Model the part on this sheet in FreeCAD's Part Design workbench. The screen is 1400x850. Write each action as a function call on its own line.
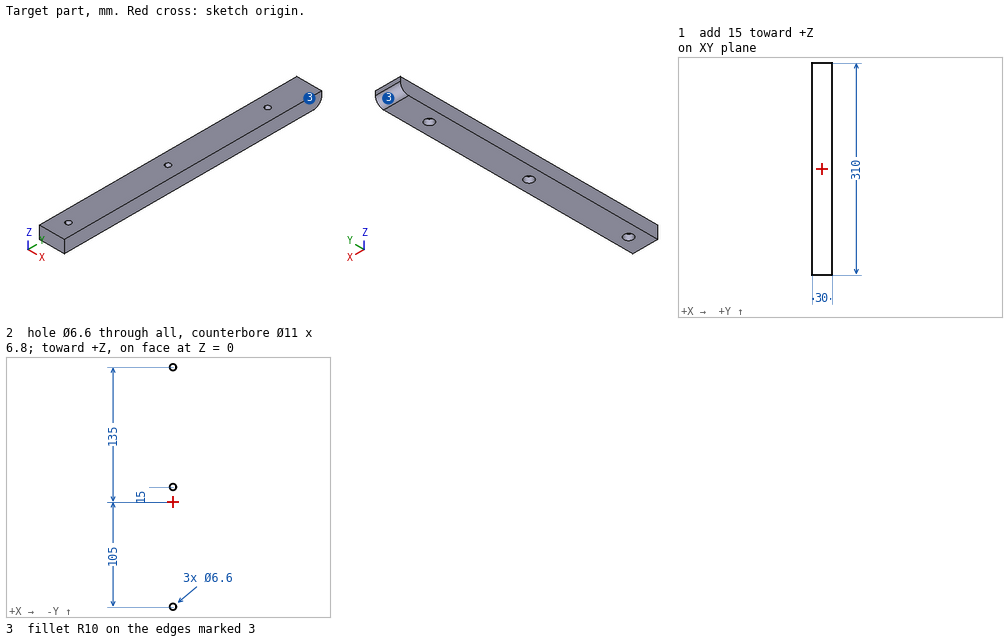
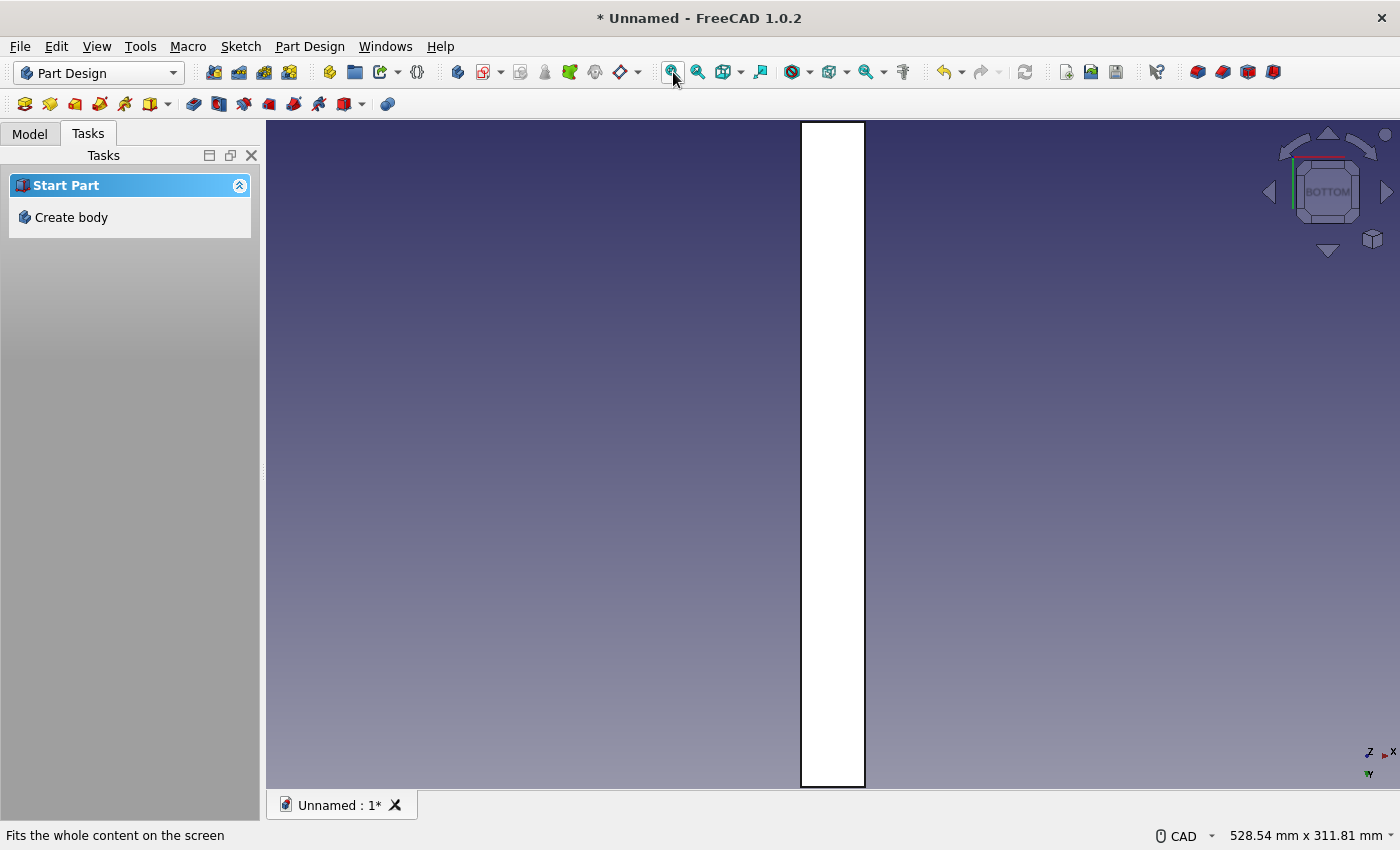
click(833, 739)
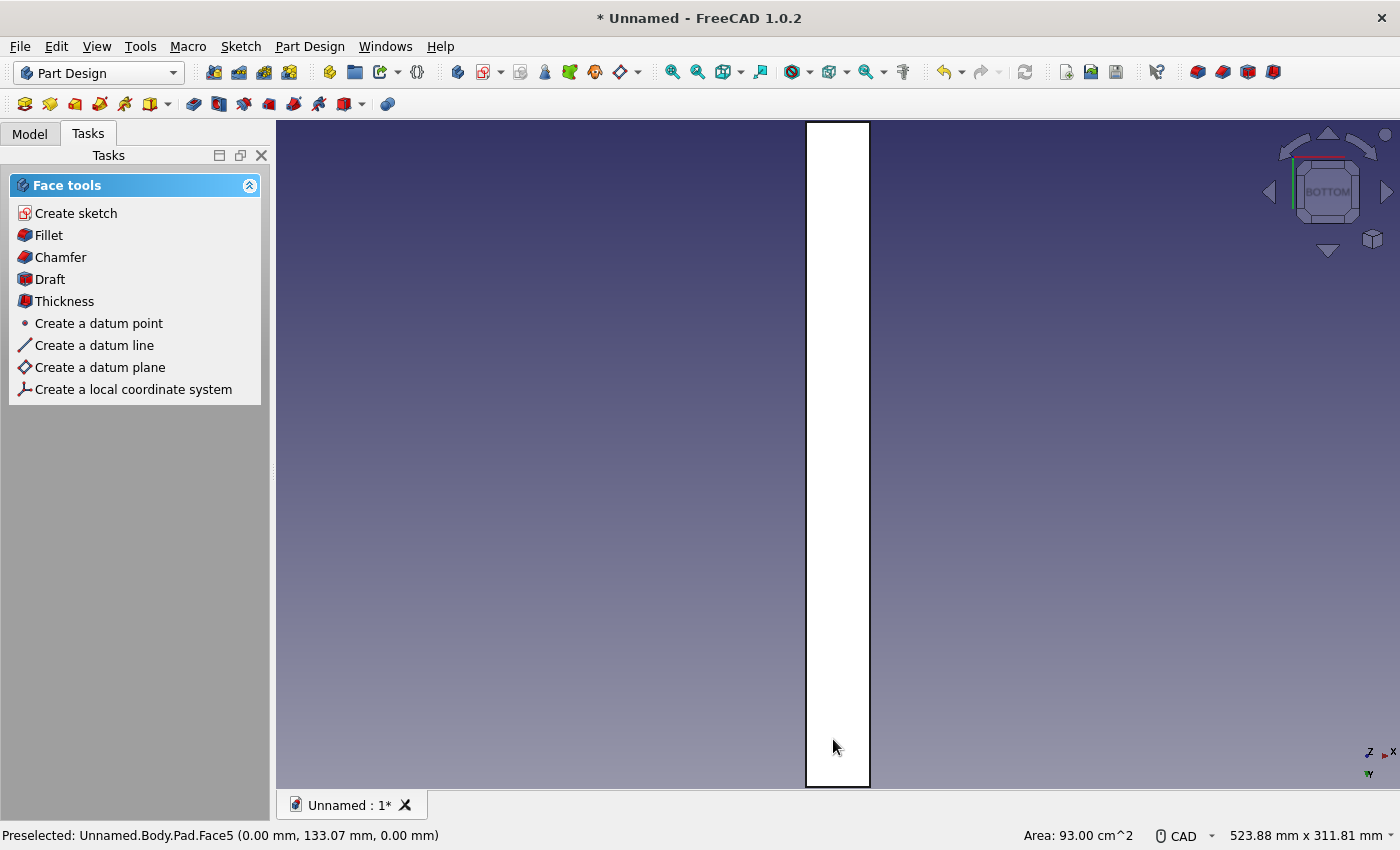
click(482, 72)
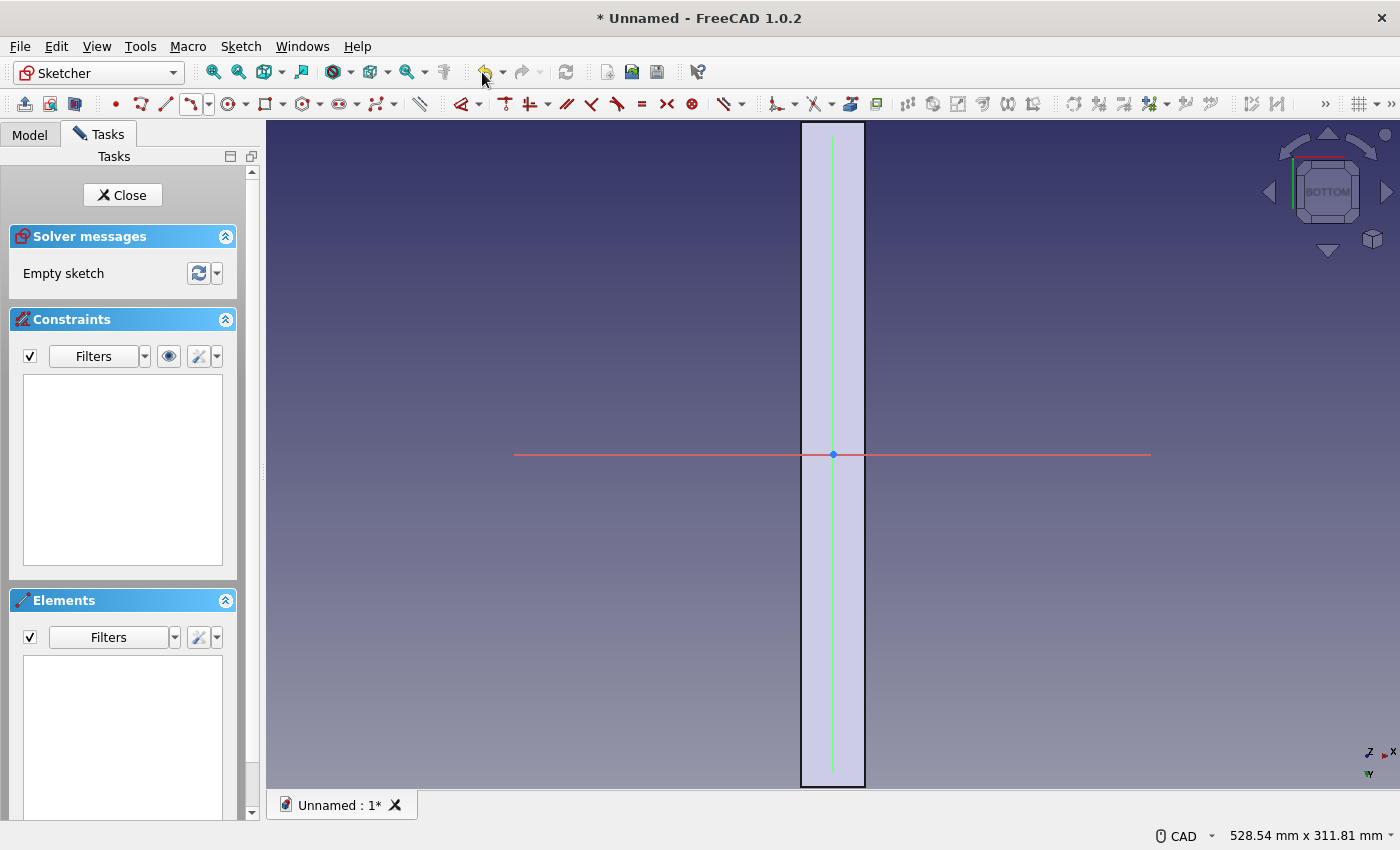
scroll(455, 600, down, 1)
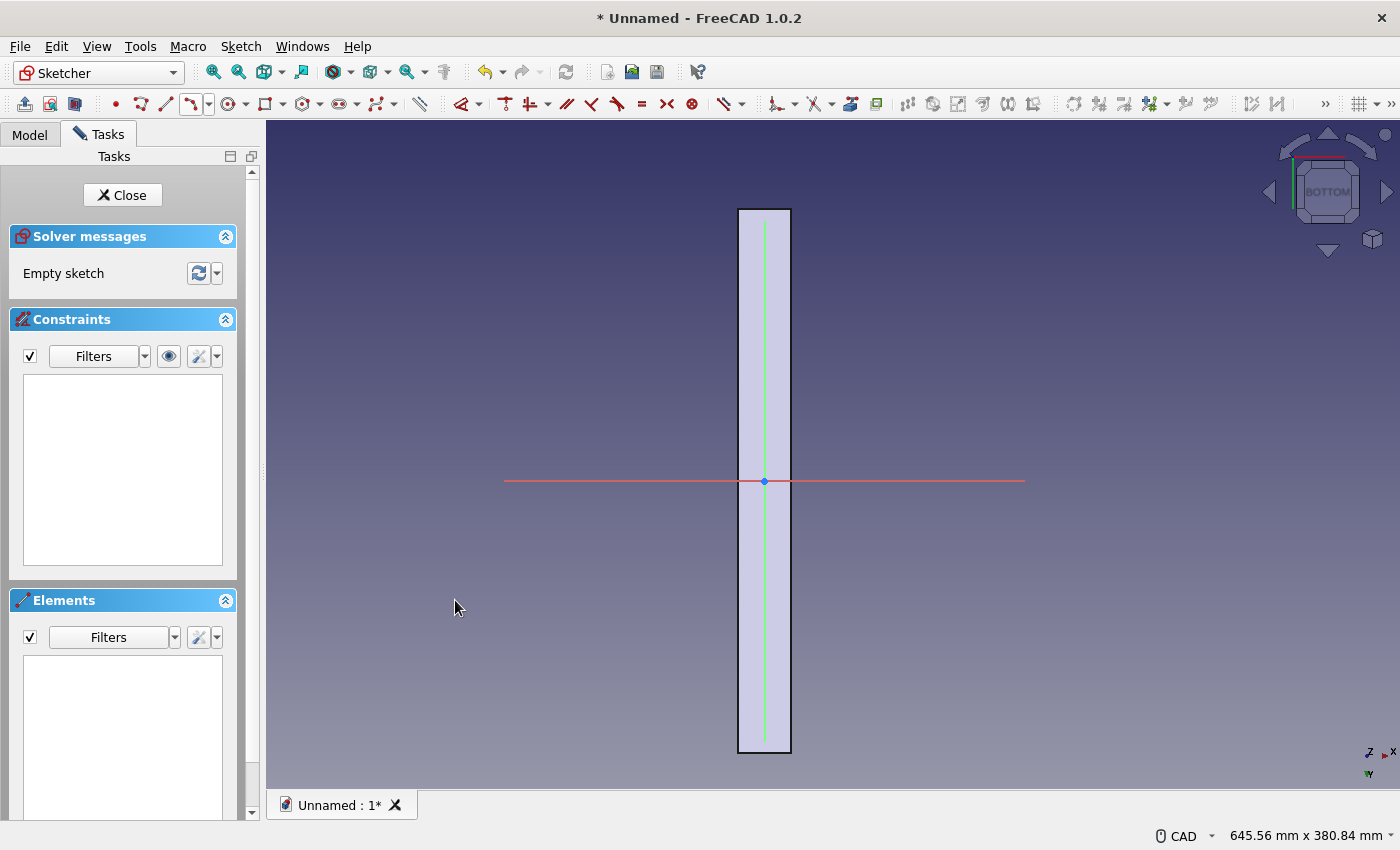
click(228, 104)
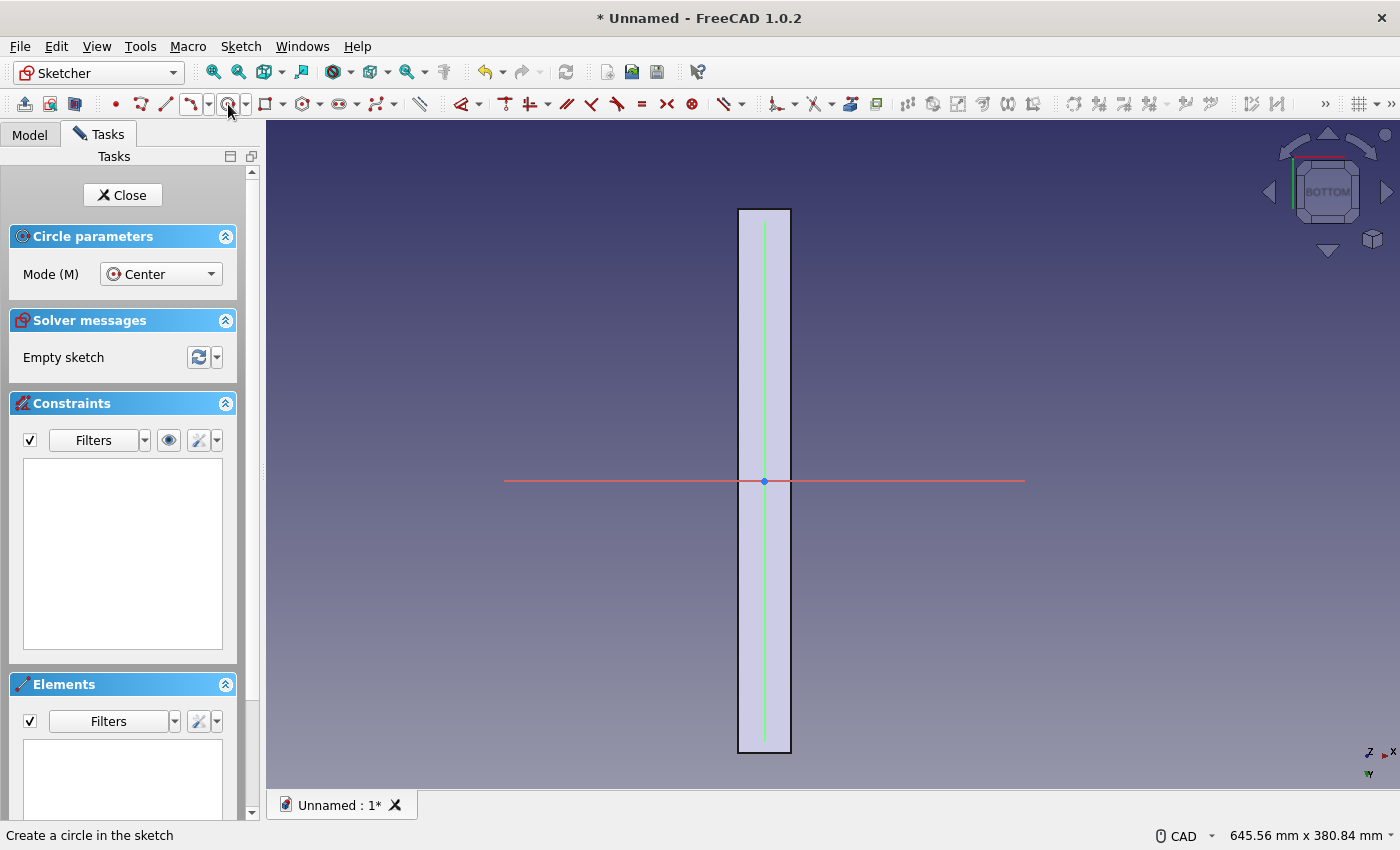
scroll(765, 665, up, 7)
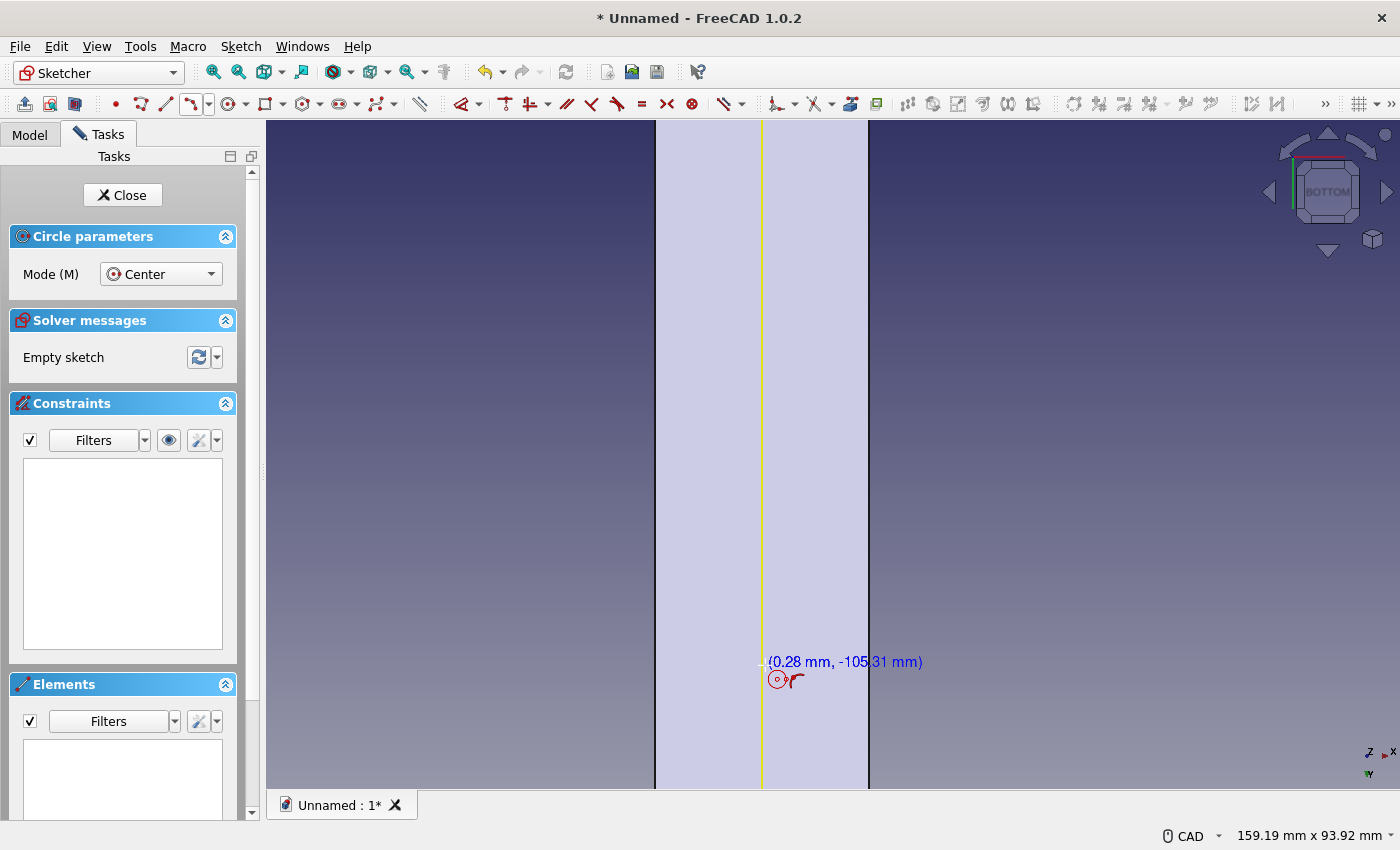
scroll(765, 666, down, 7)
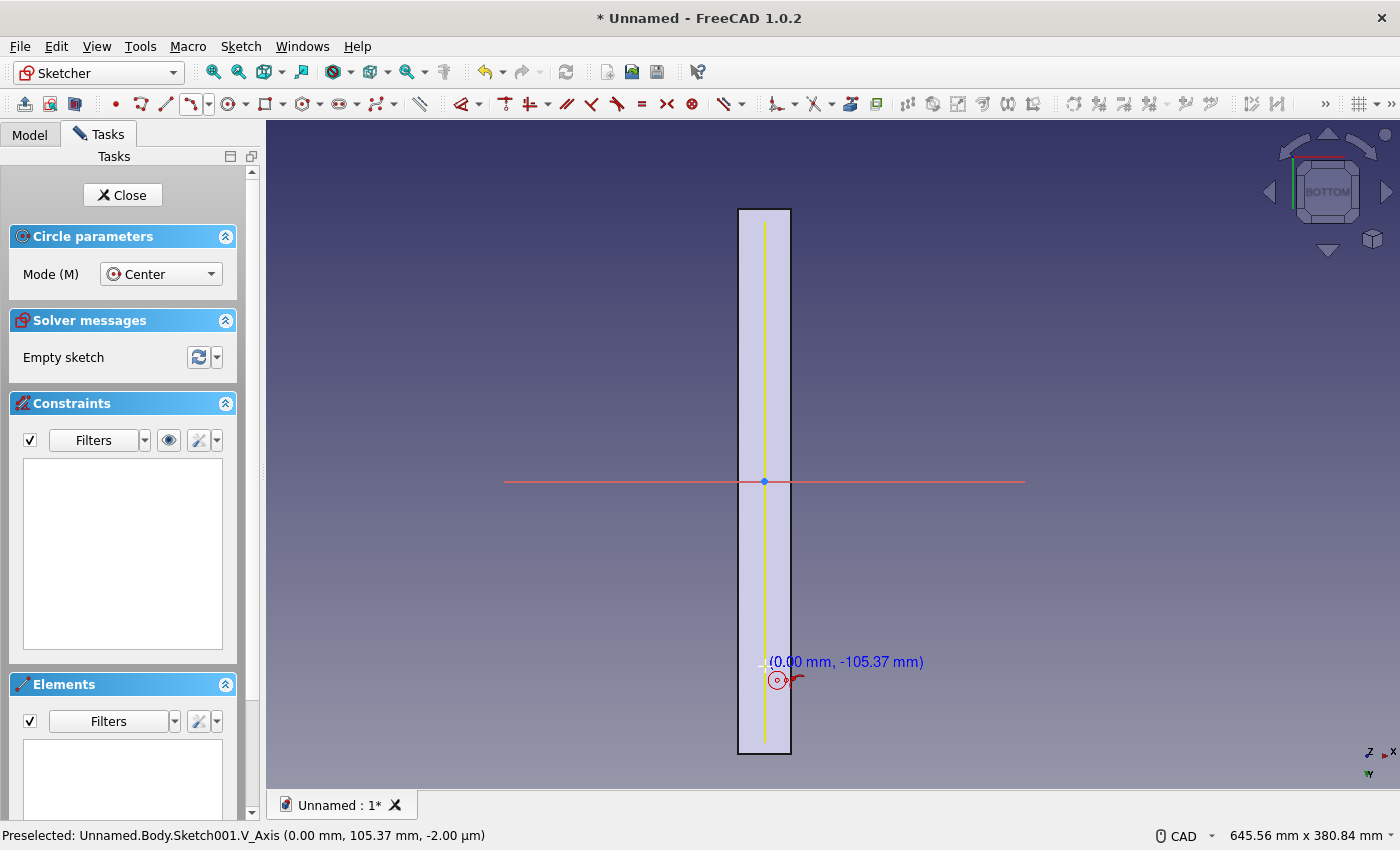
click(765, 666)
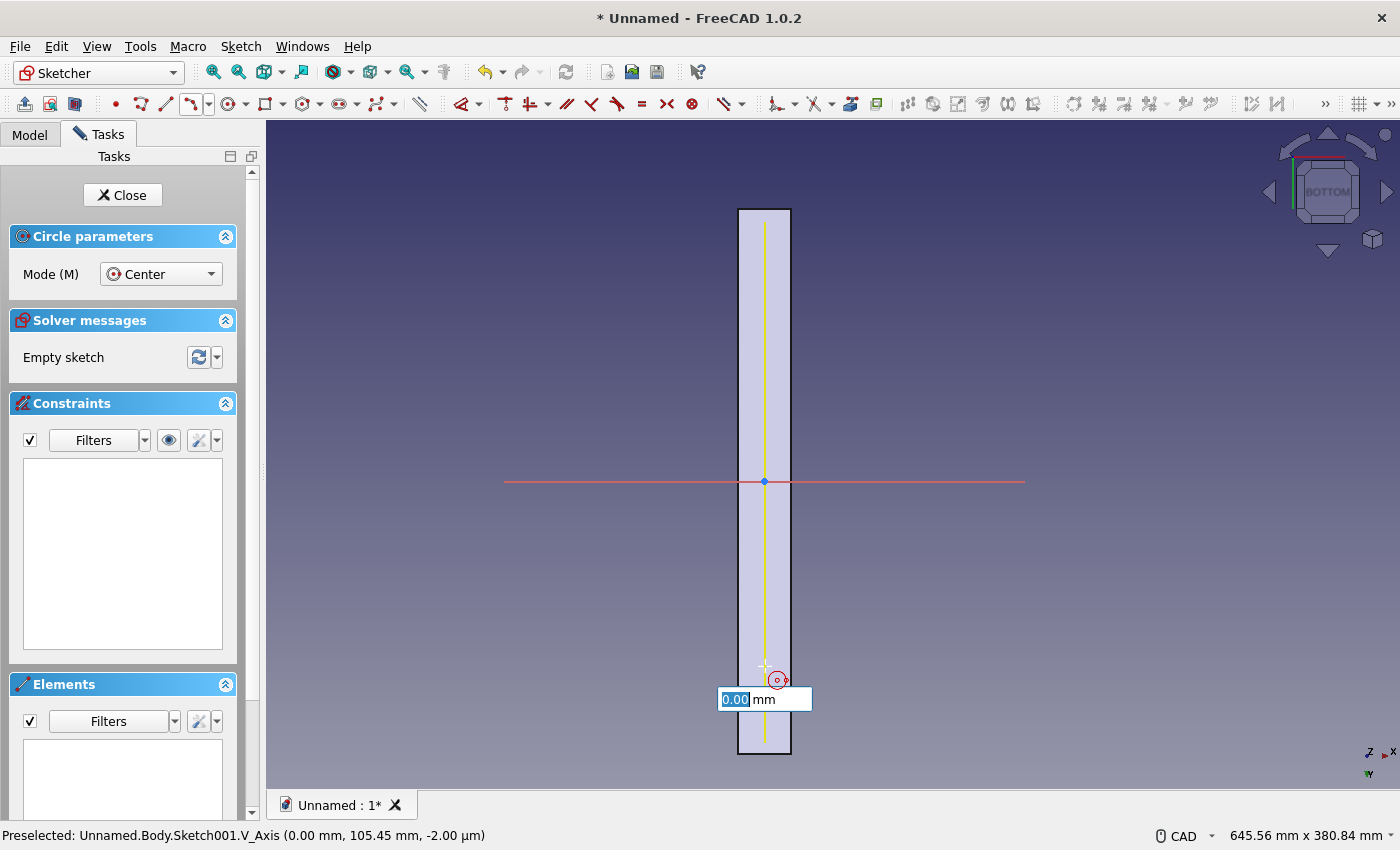
scroll(770, 664, up, 6)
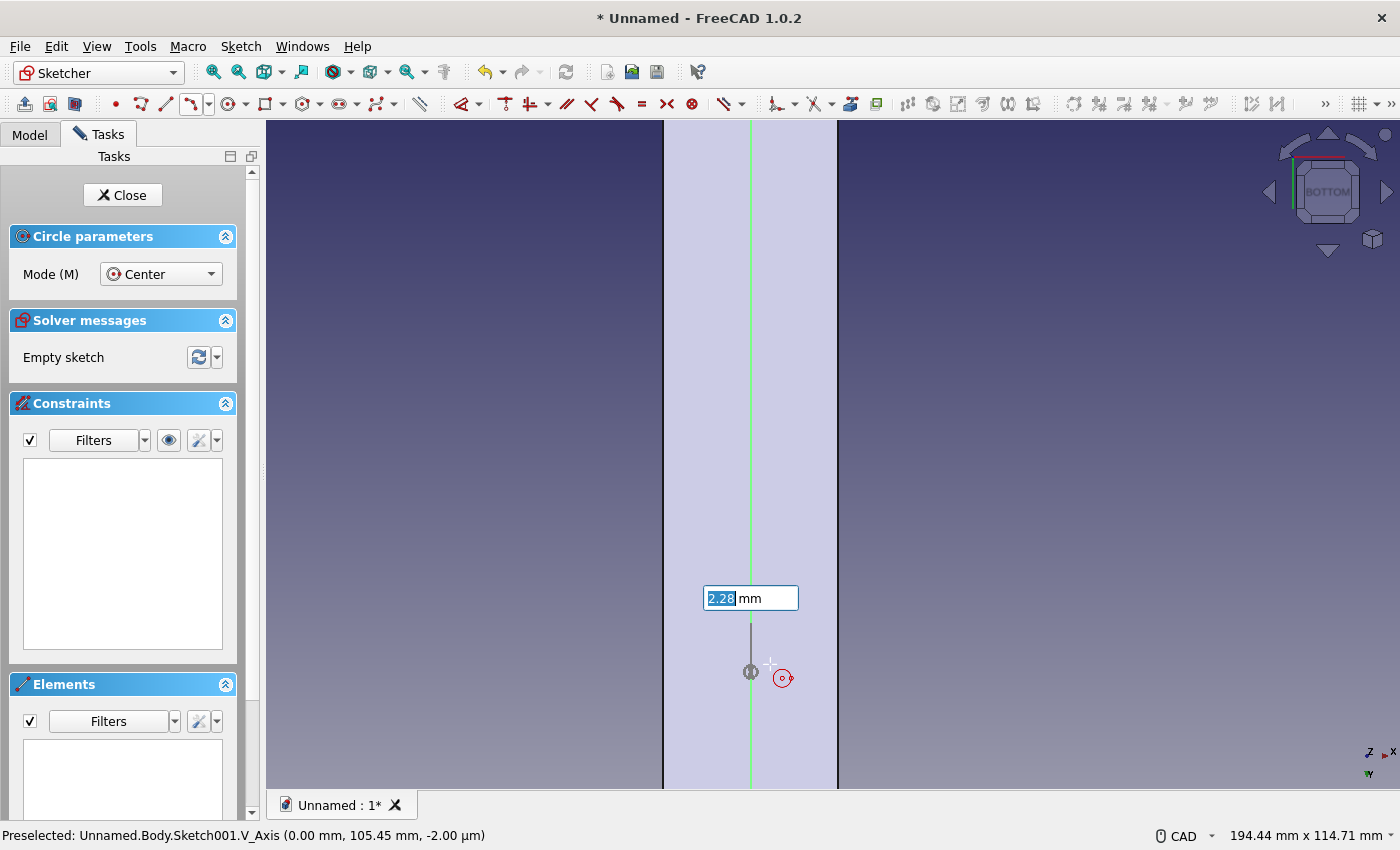
click(769, 663)